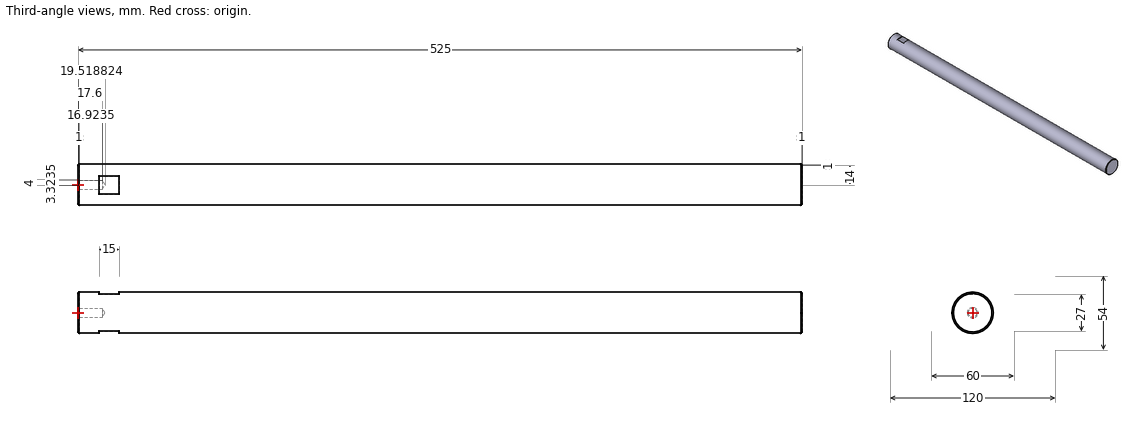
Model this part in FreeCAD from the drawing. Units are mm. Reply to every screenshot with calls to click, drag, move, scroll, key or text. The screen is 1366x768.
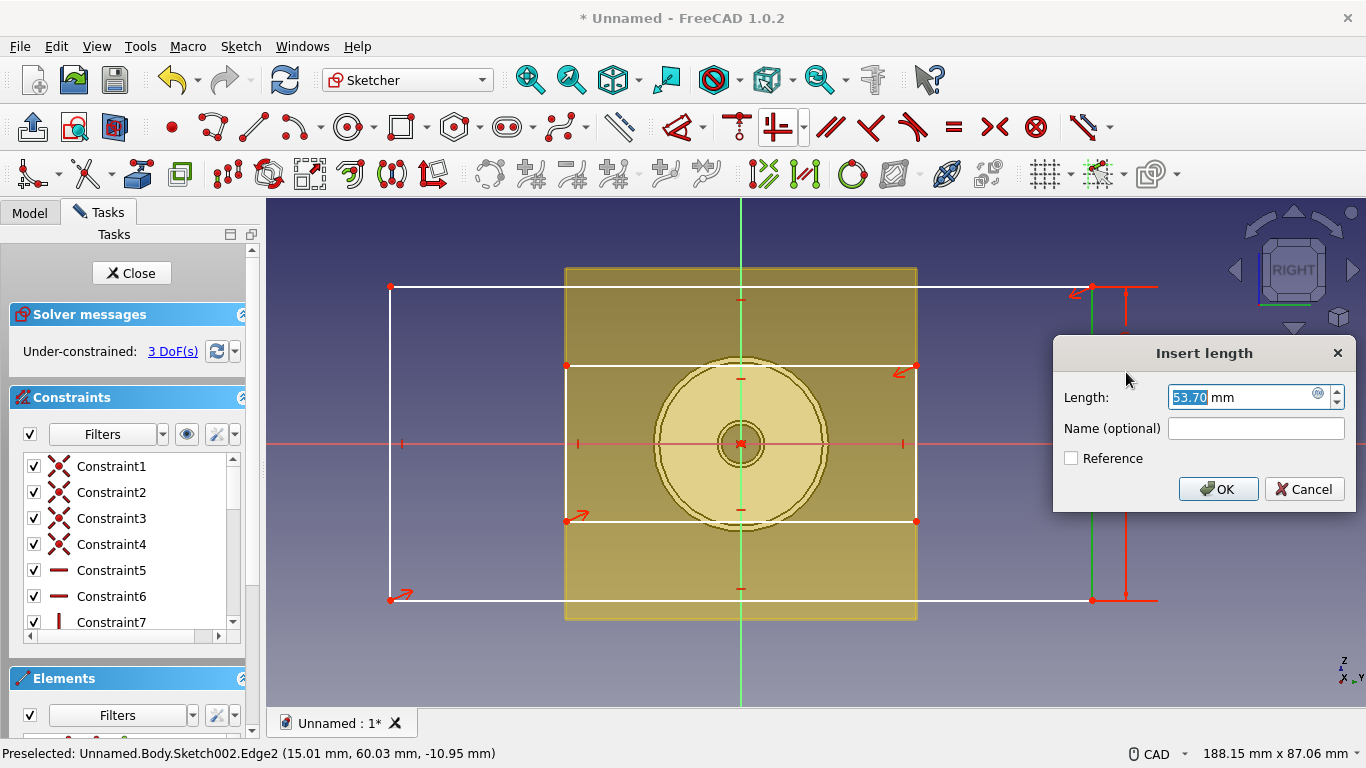
text(54)
key(Return)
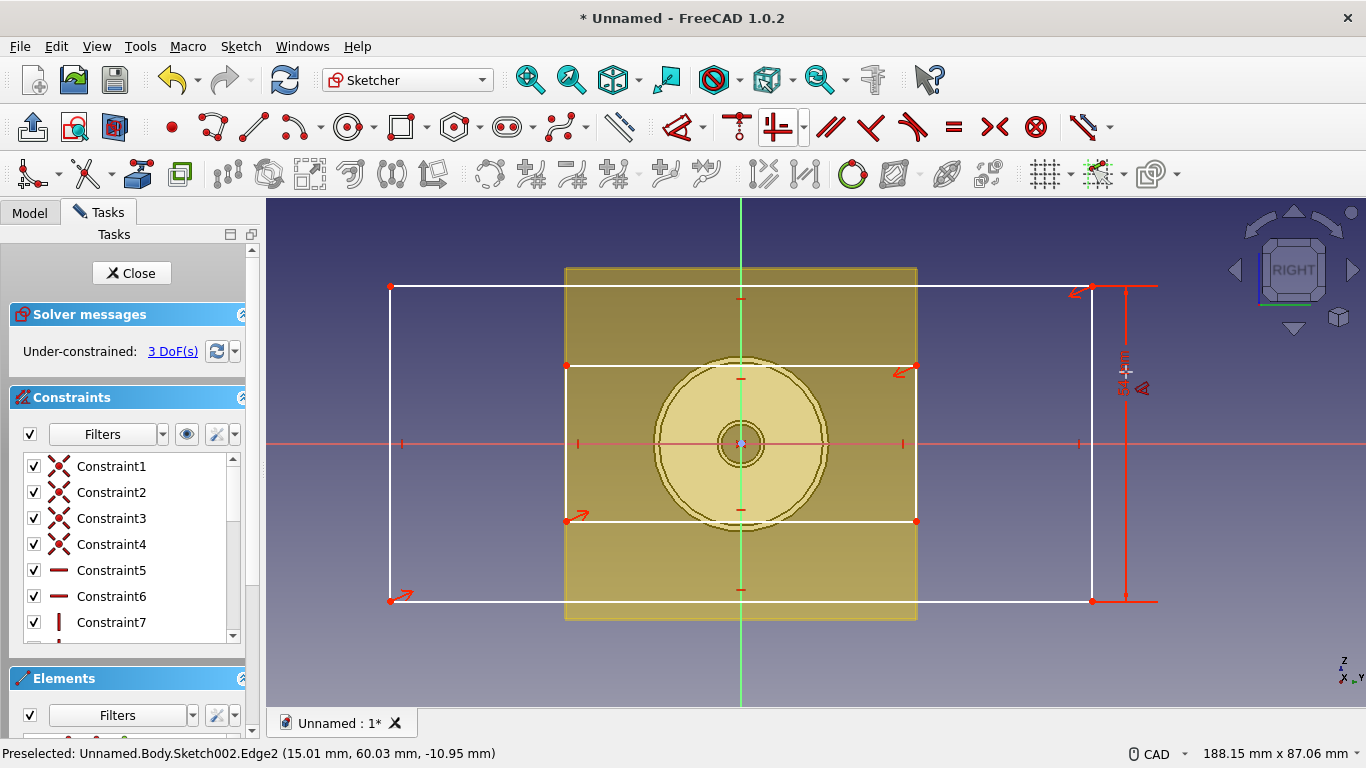
click(671, 522)
click(661, 556)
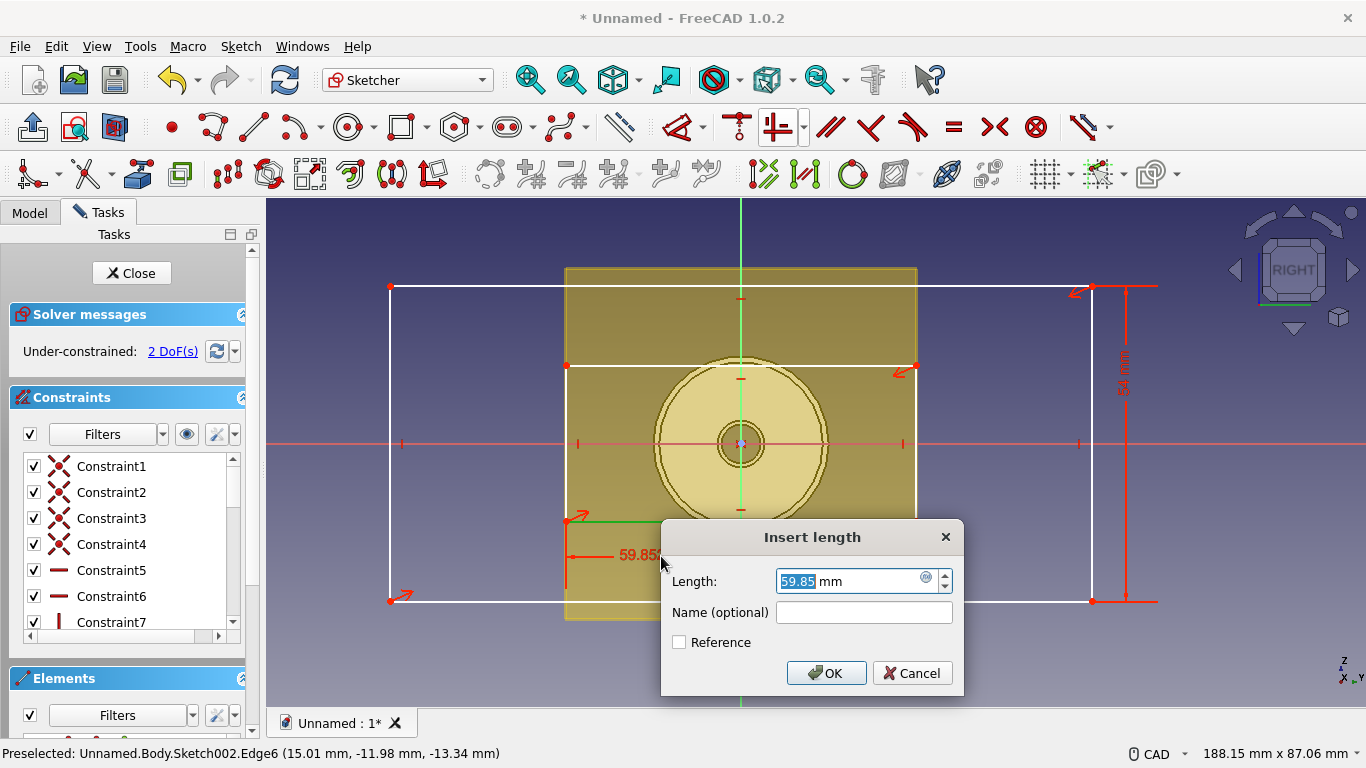
text(60)
key(Return)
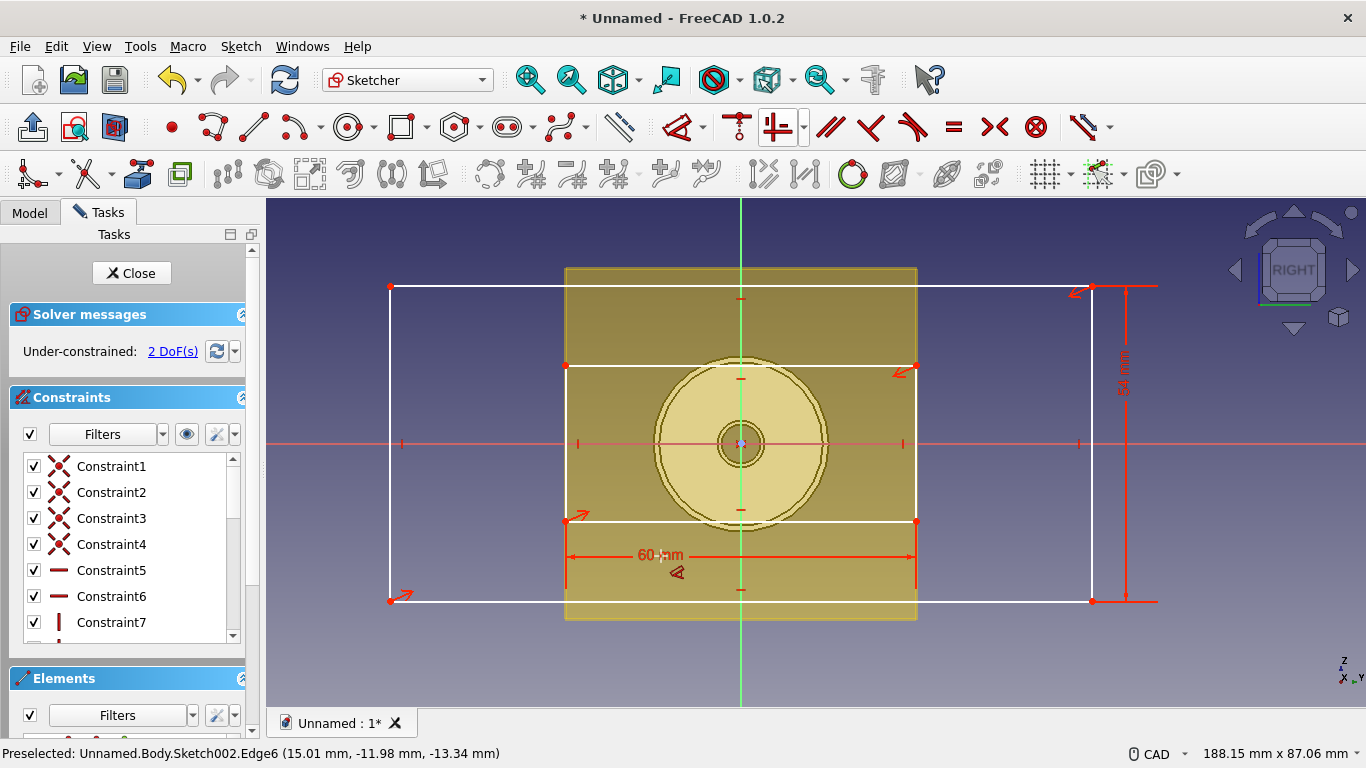
click(916, 475)
click(950, 408)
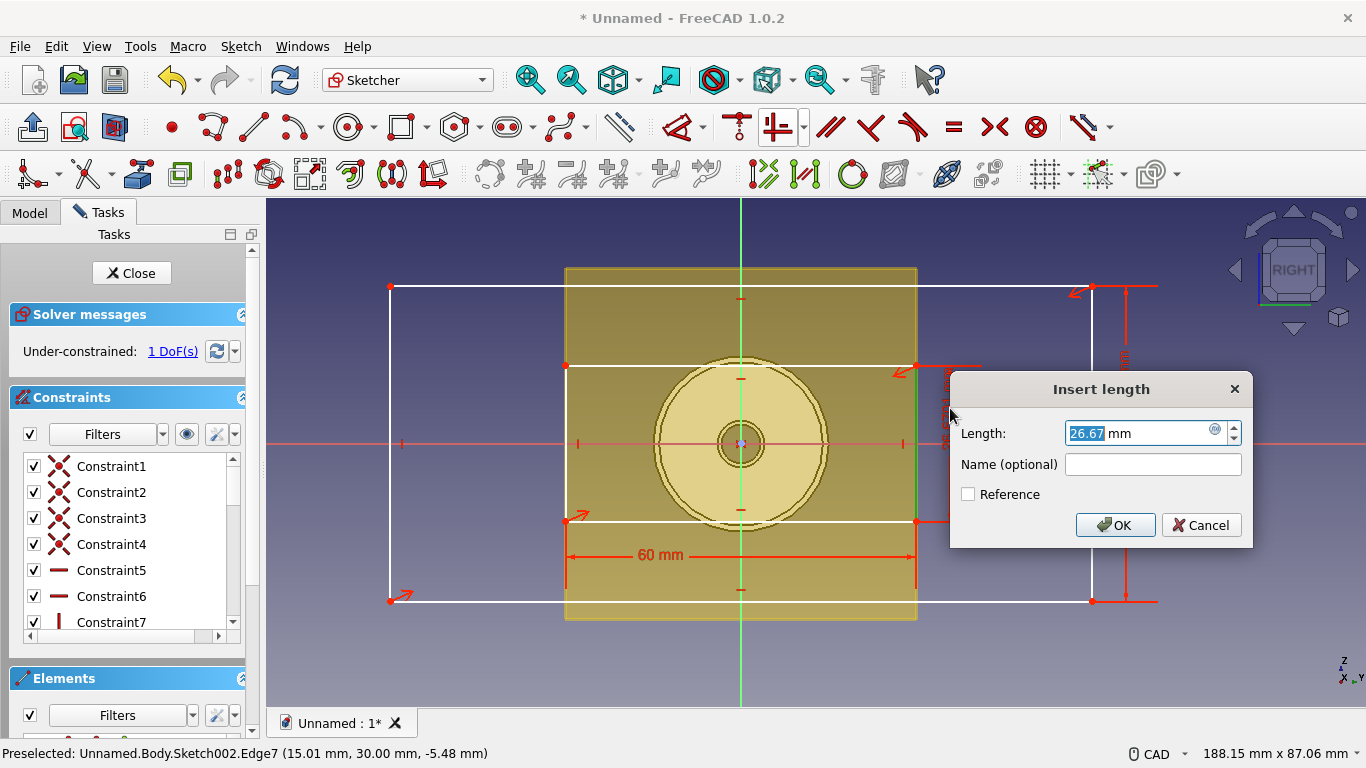
text(27)
key(Return)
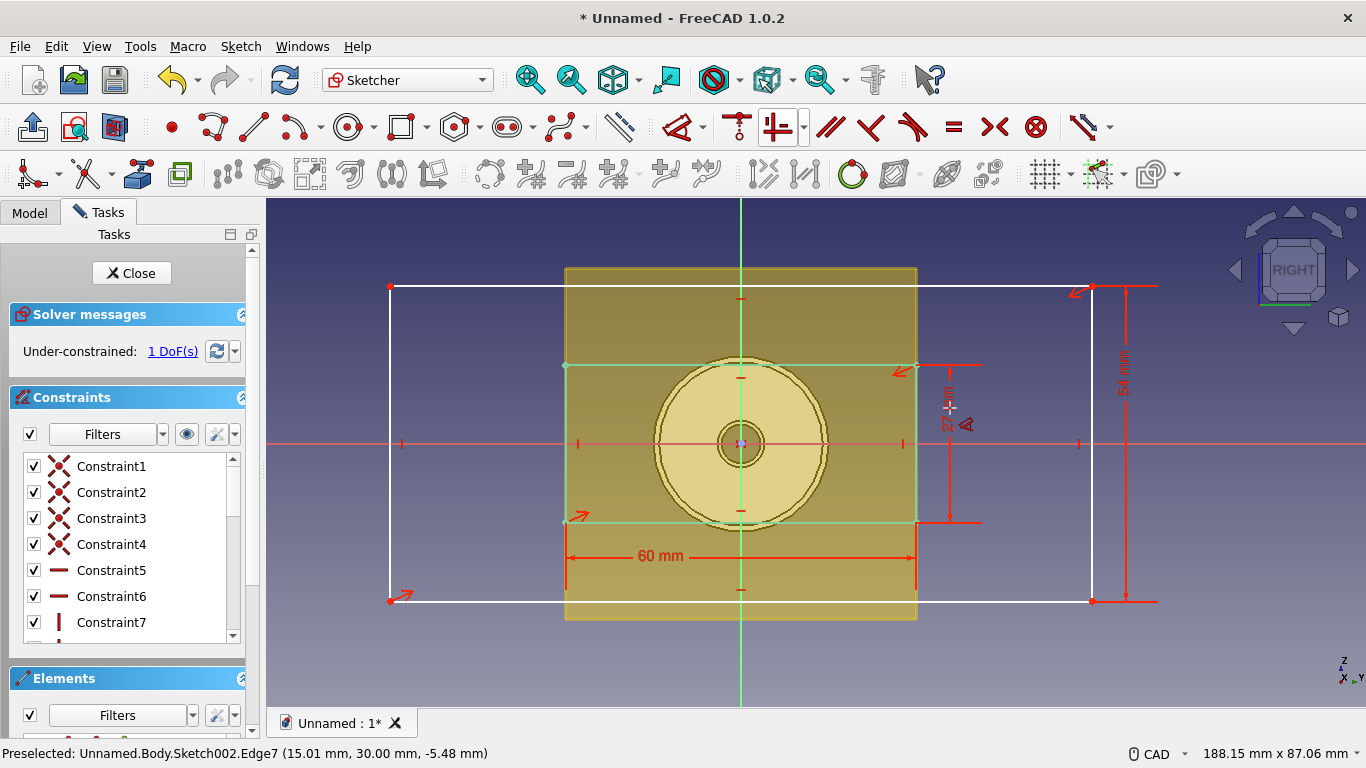
click(601, 602)
click(580, 636)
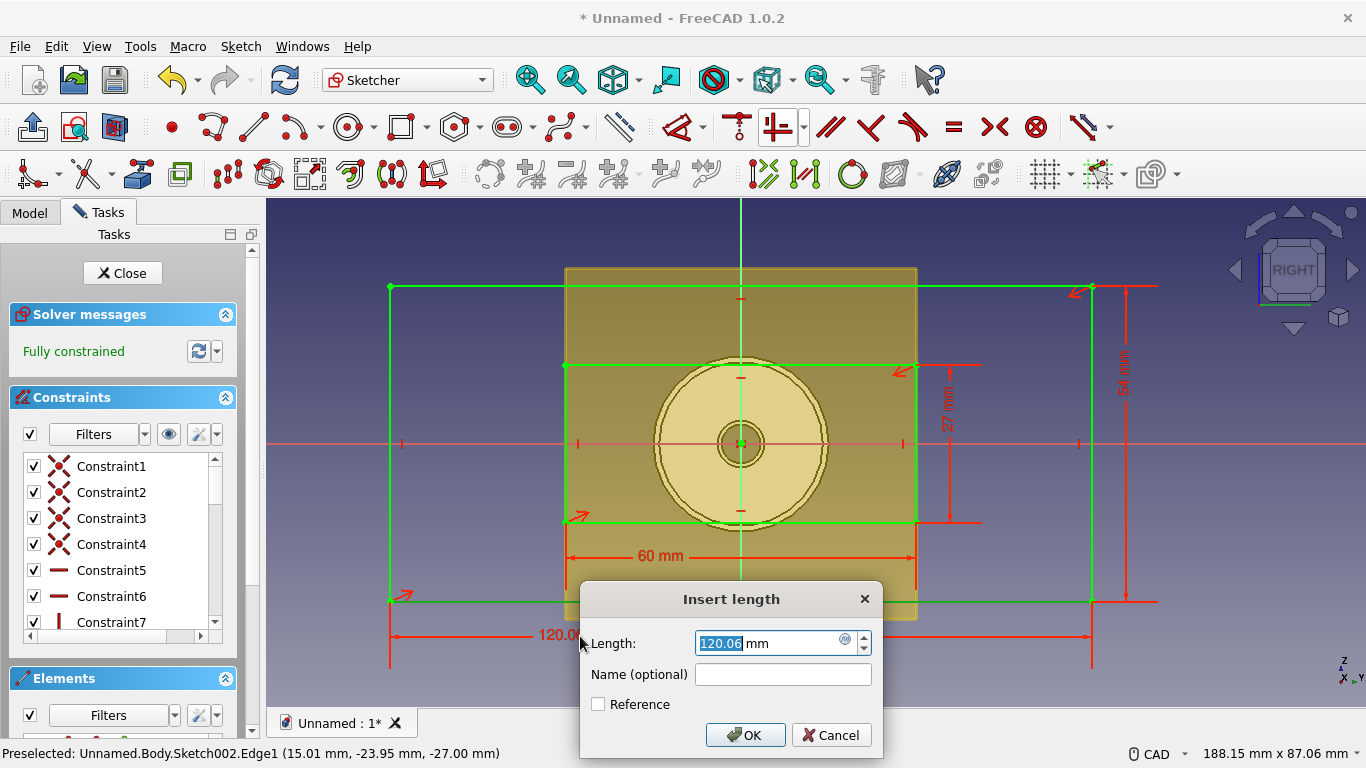
text(120)
key(Return)
key(Escape)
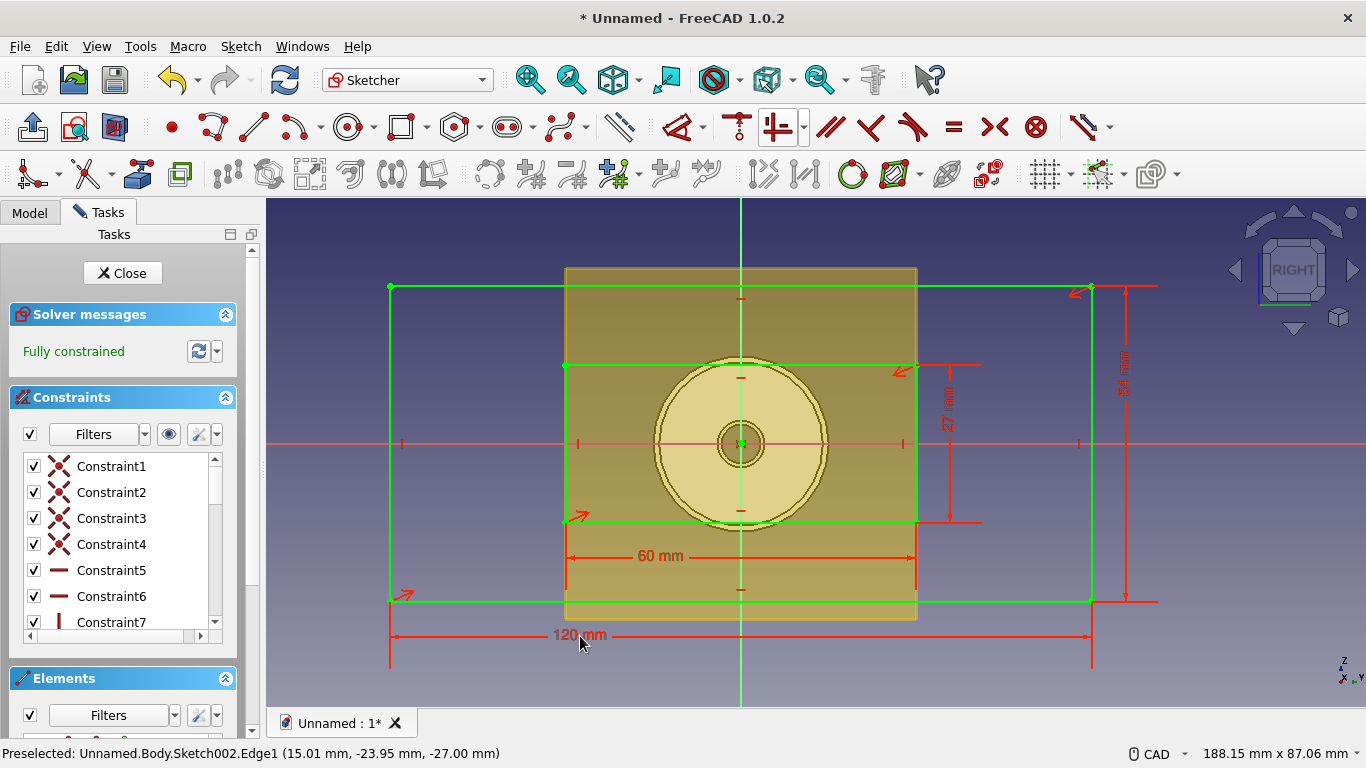
click(123, 273)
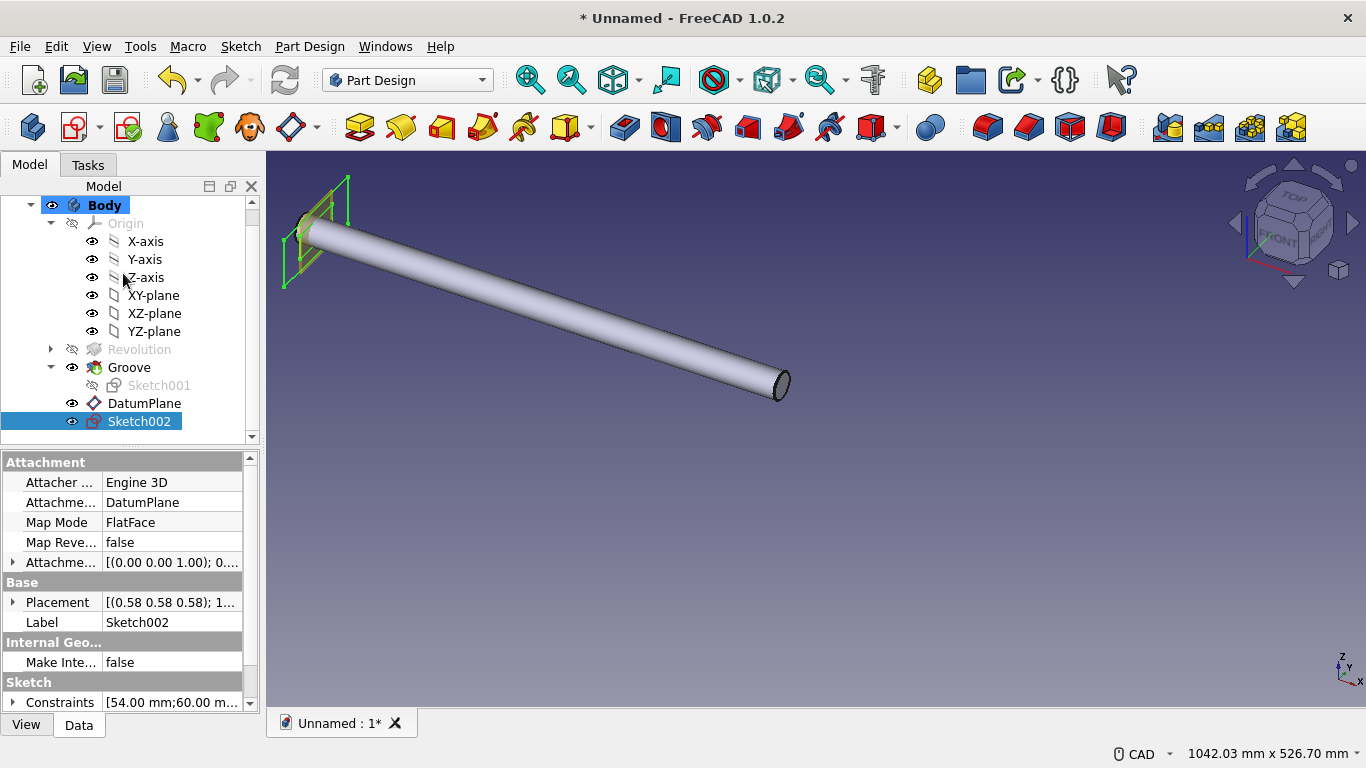
click(625, 128)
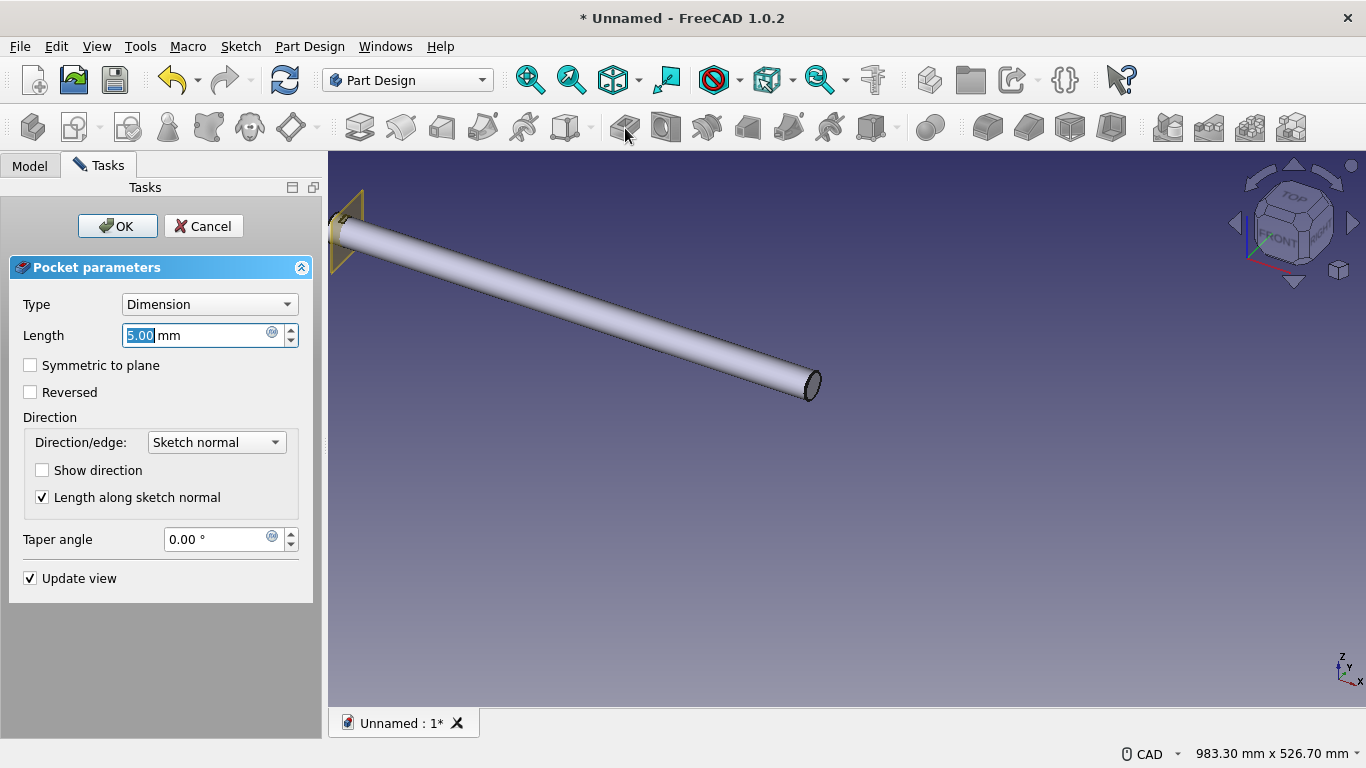
text(15)
key(Tab)